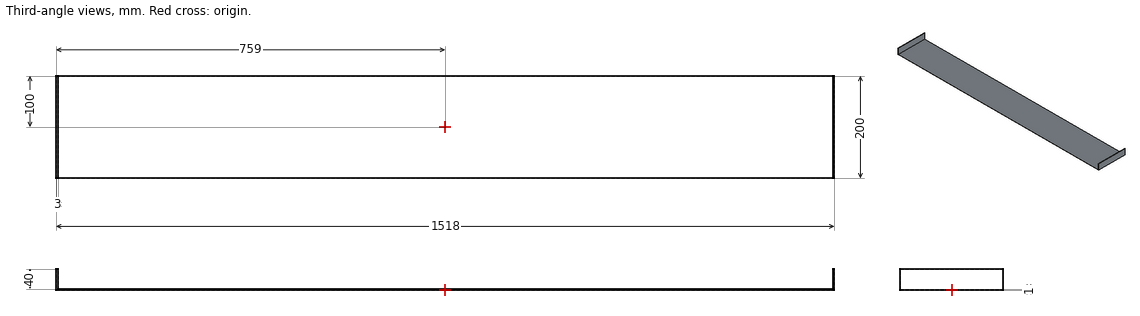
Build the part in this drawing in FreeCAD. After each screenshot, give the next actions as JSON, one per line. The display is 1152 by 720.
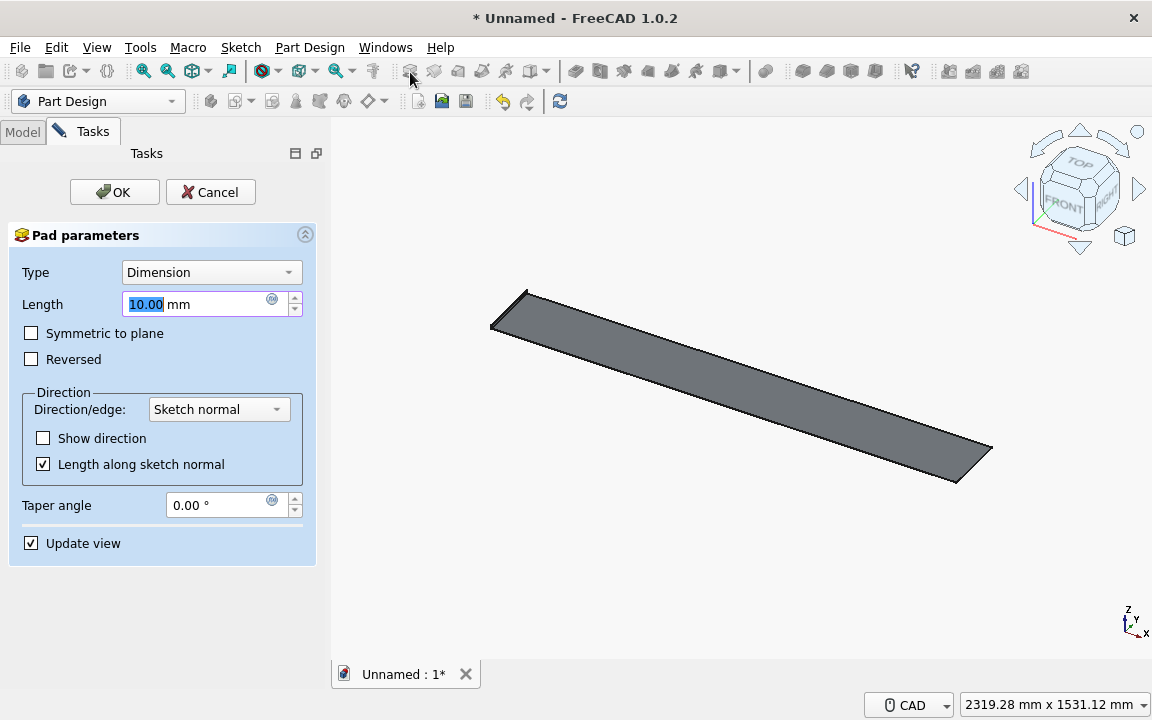
{"action": "type", "text": "40"}
{"action": "key", "text": "Tab"}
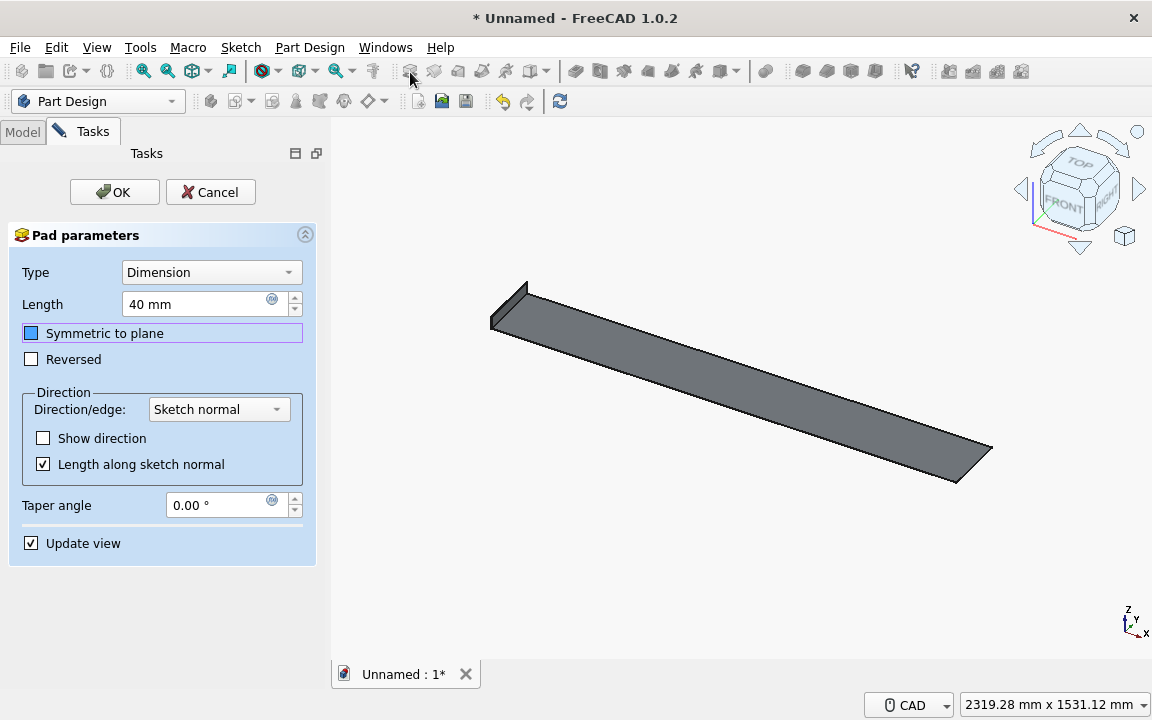
{"action": "left_click", "coordinate": [115, 192]}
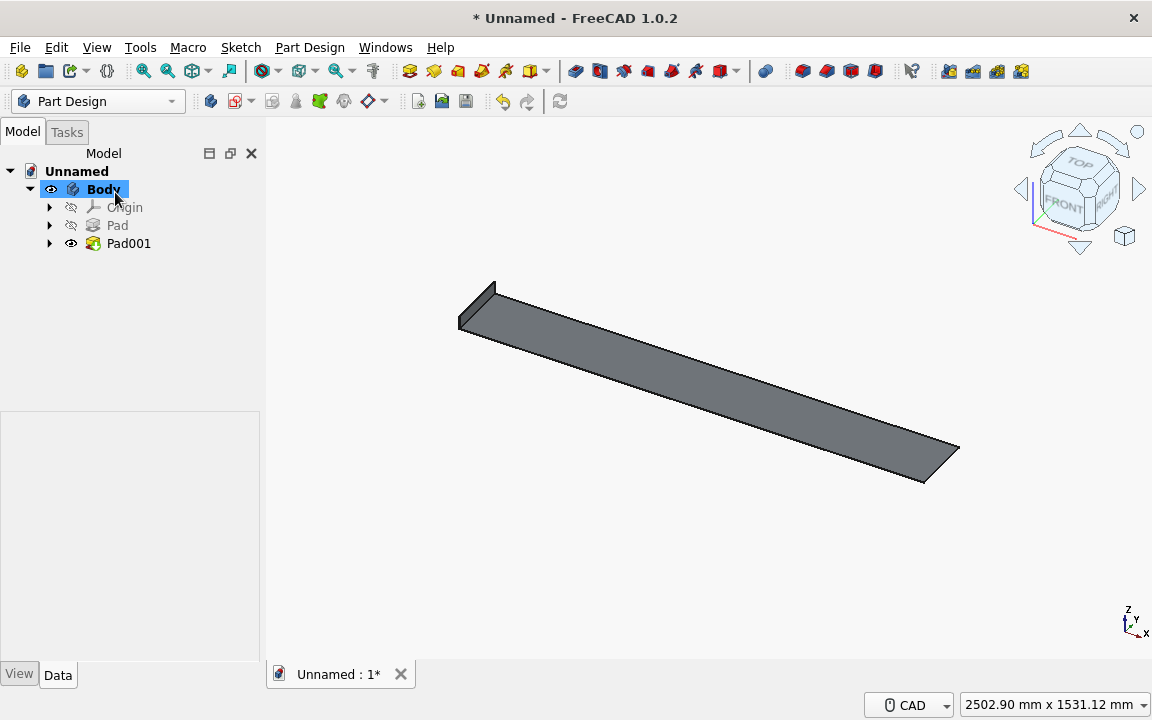
{"action": "left_click", "coordinate": [116, 243]}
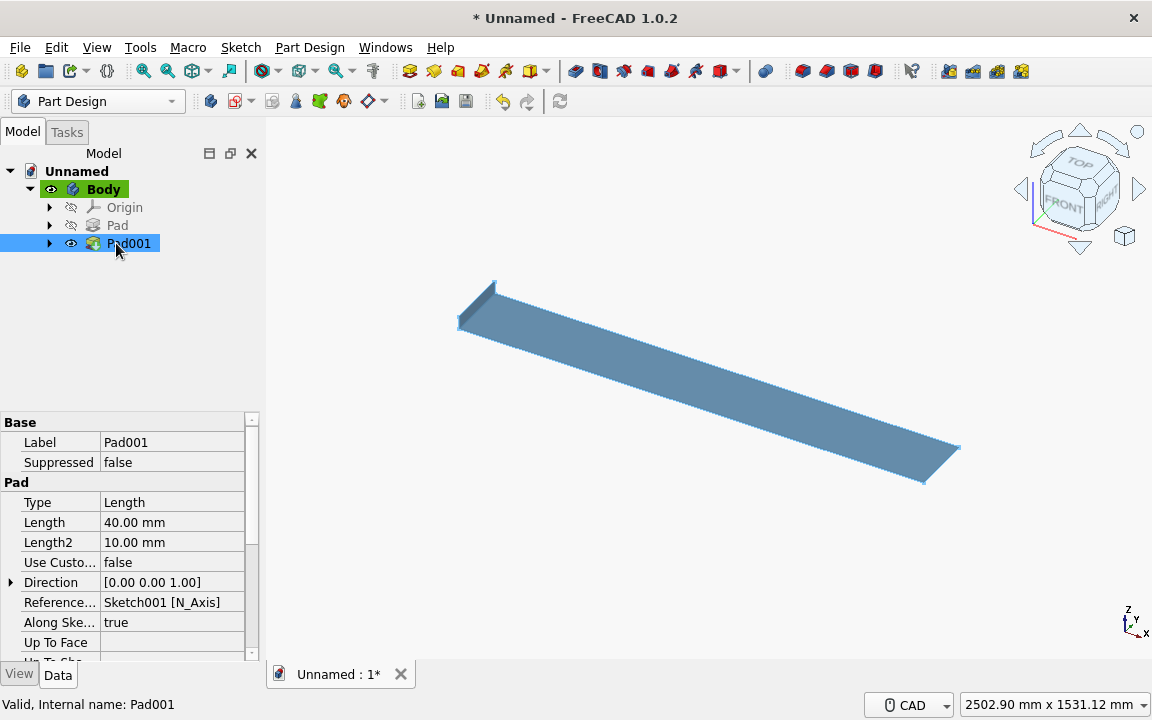
{"action": "left_click", "coordinate": [950, 72]}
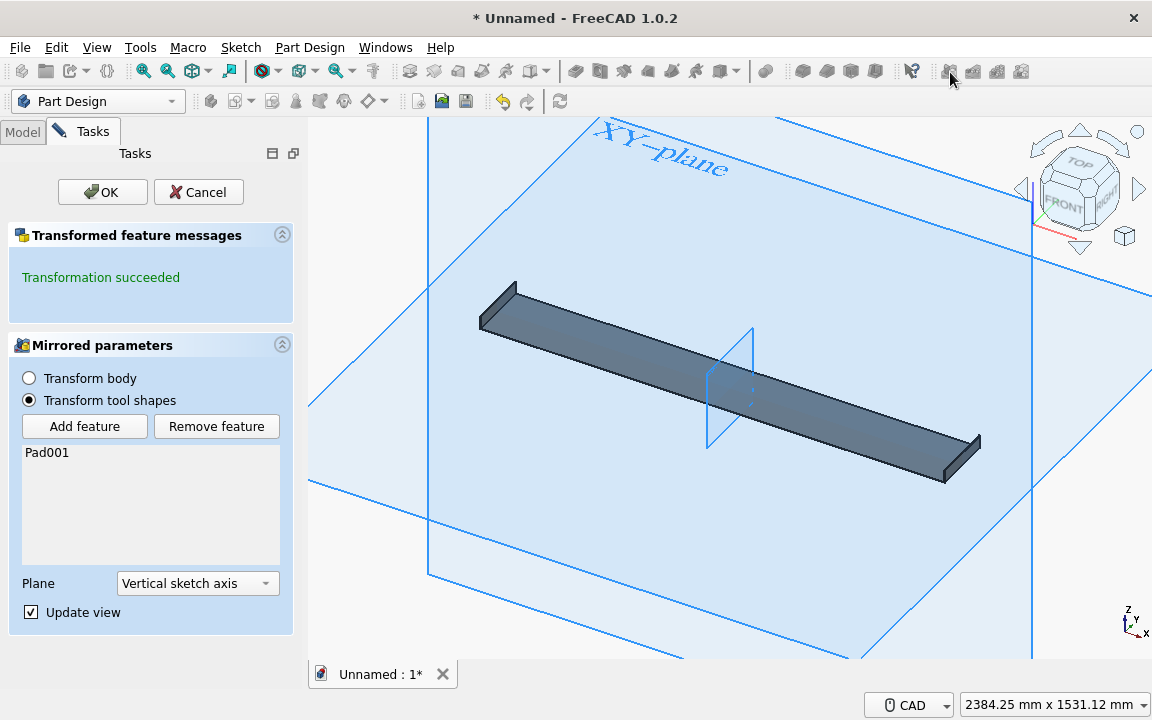
{"action": "left_click", "coordinate": [198, 584]}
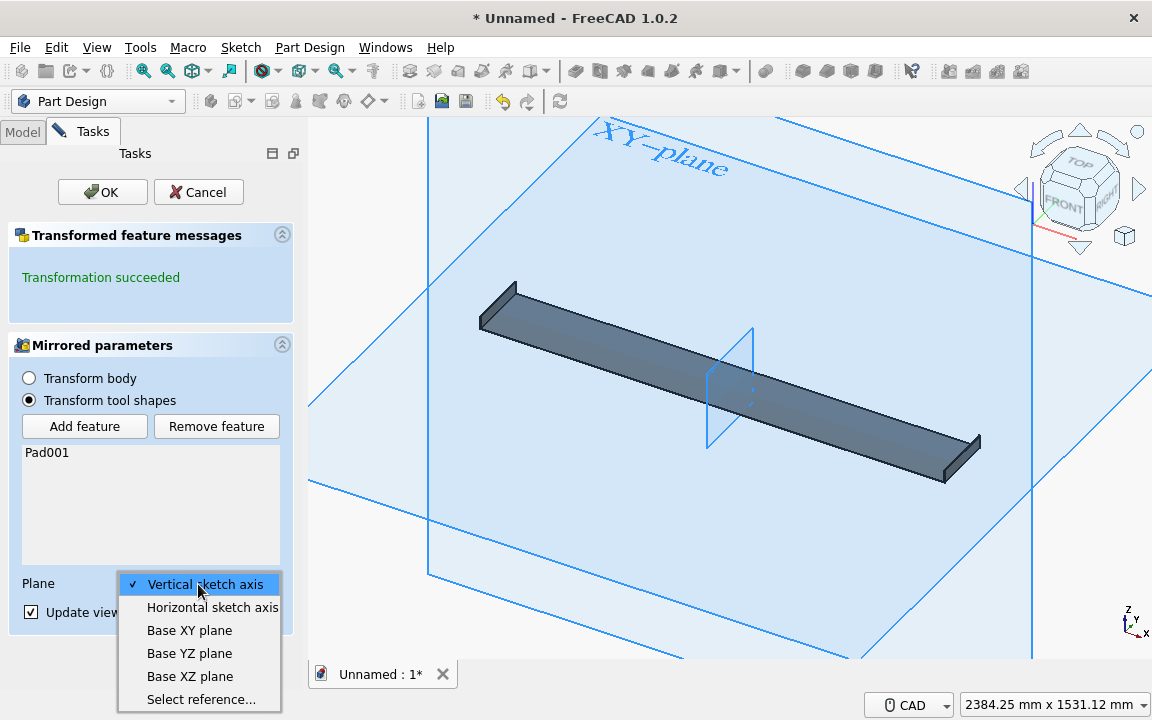
{"action": "left_click", "coordinate": [198, 654]}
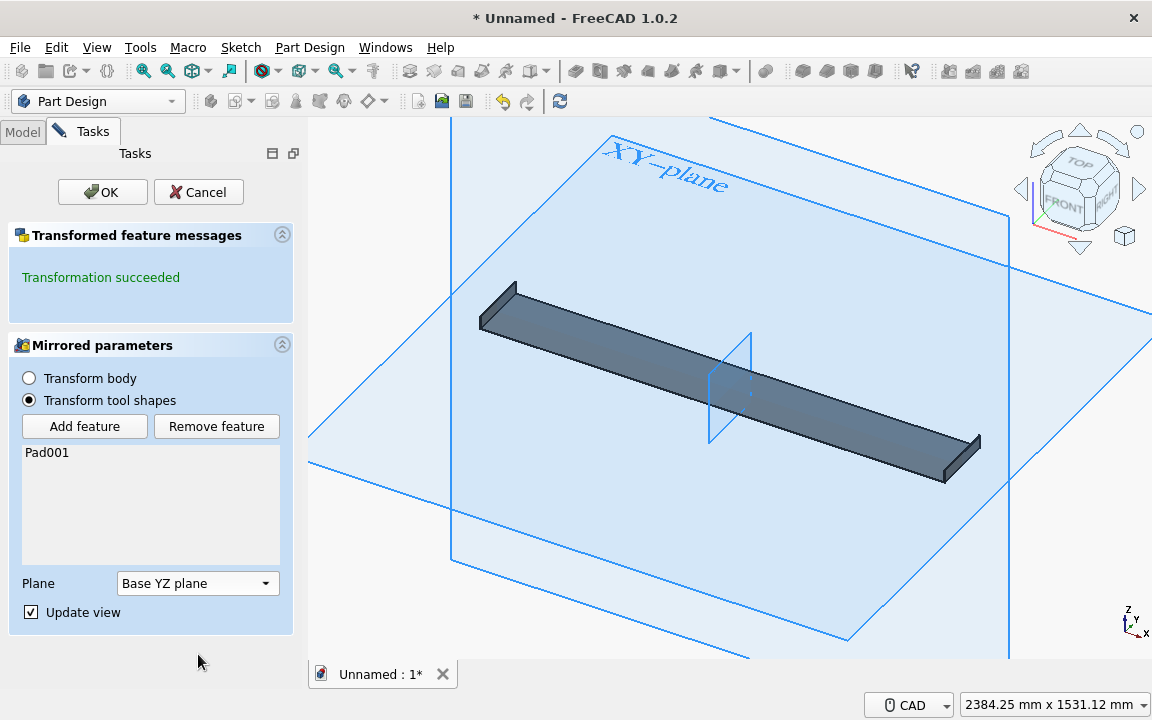
{"action": "left_click", "coordinate": [103, 192]}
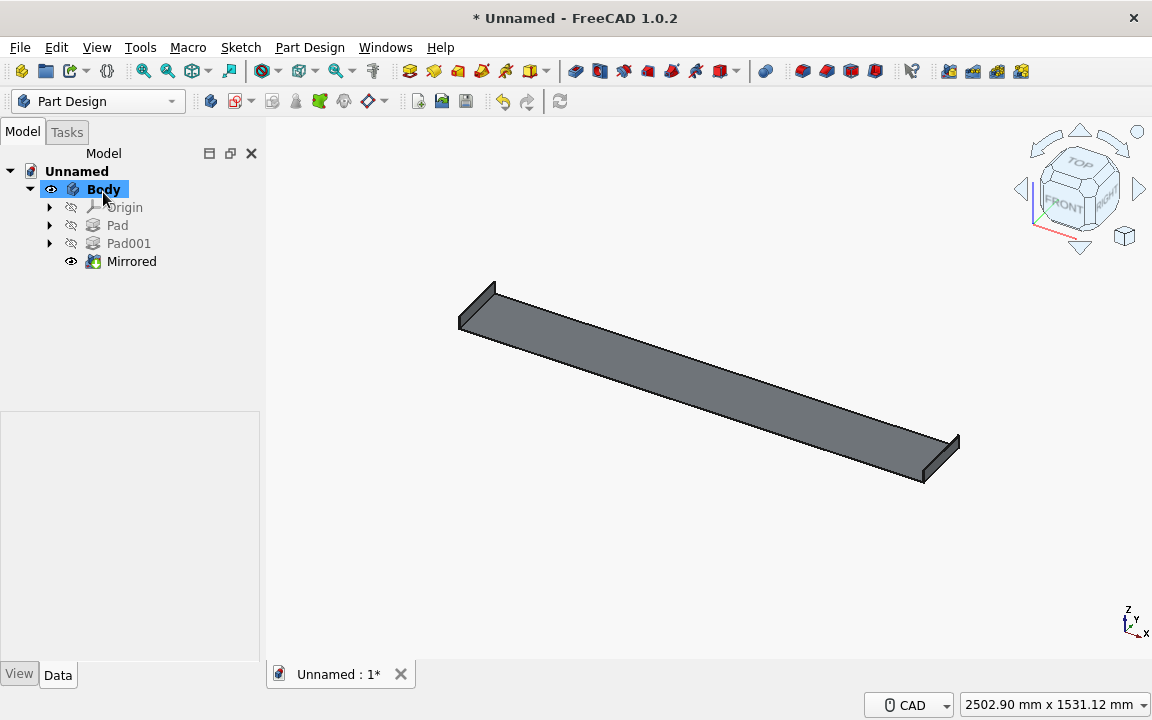
{"action": "key", "text": "0"}